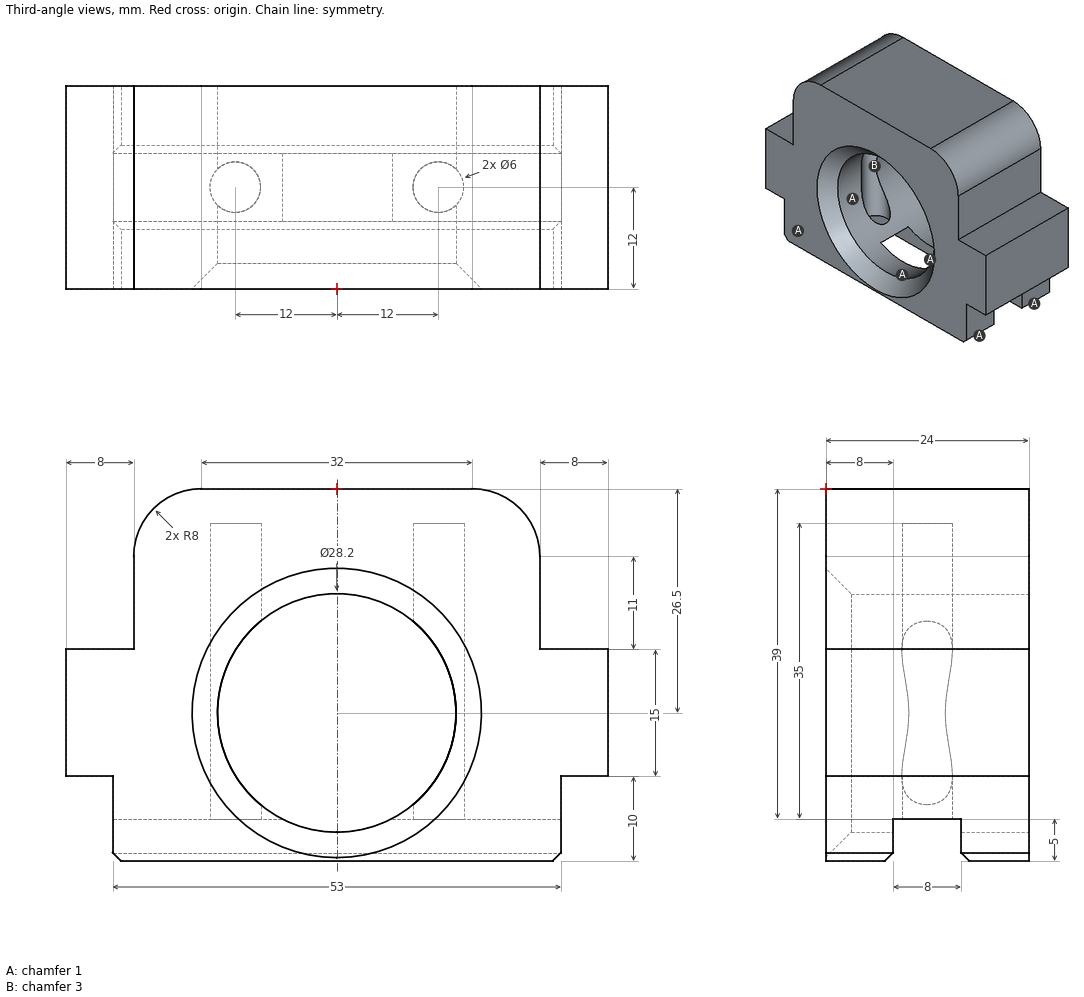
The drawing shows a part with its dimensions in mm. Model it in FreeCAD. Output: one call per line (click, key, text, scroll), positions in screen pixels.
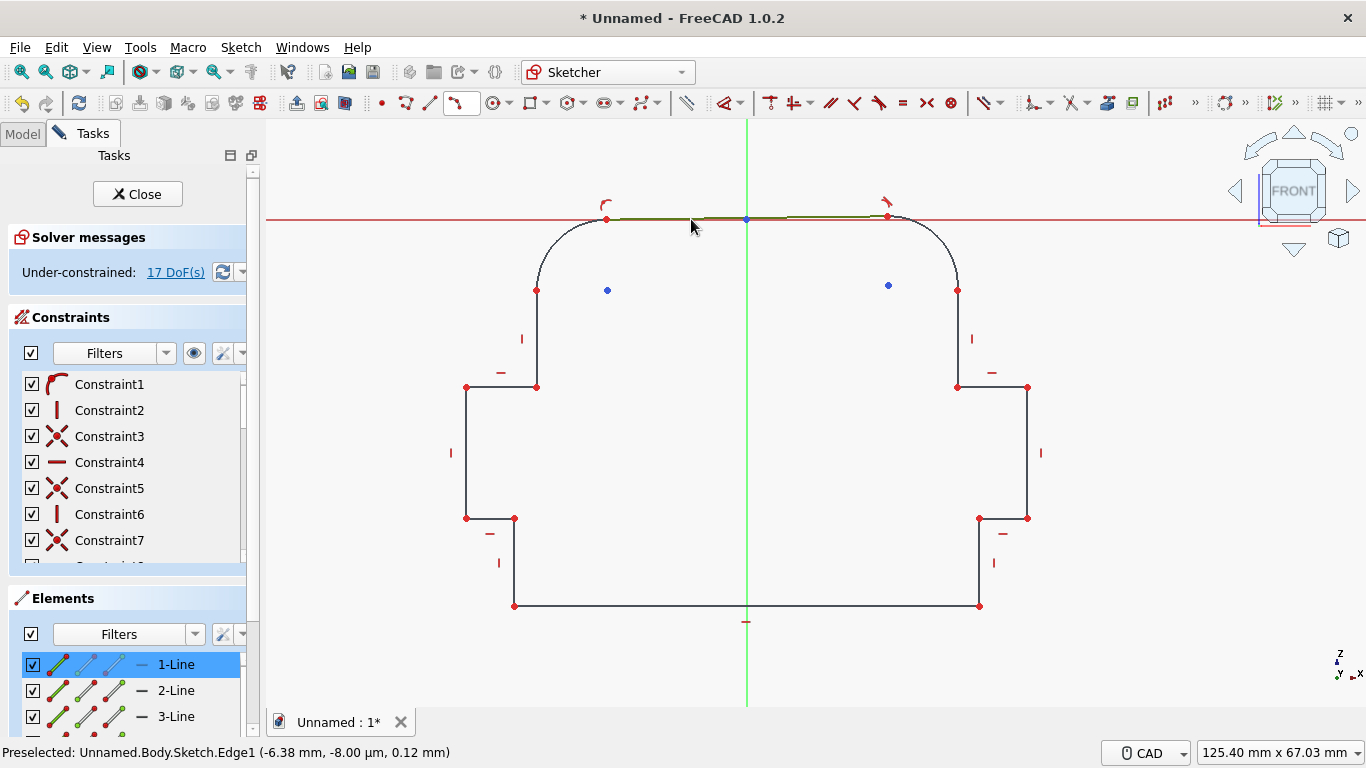
click(544, 259)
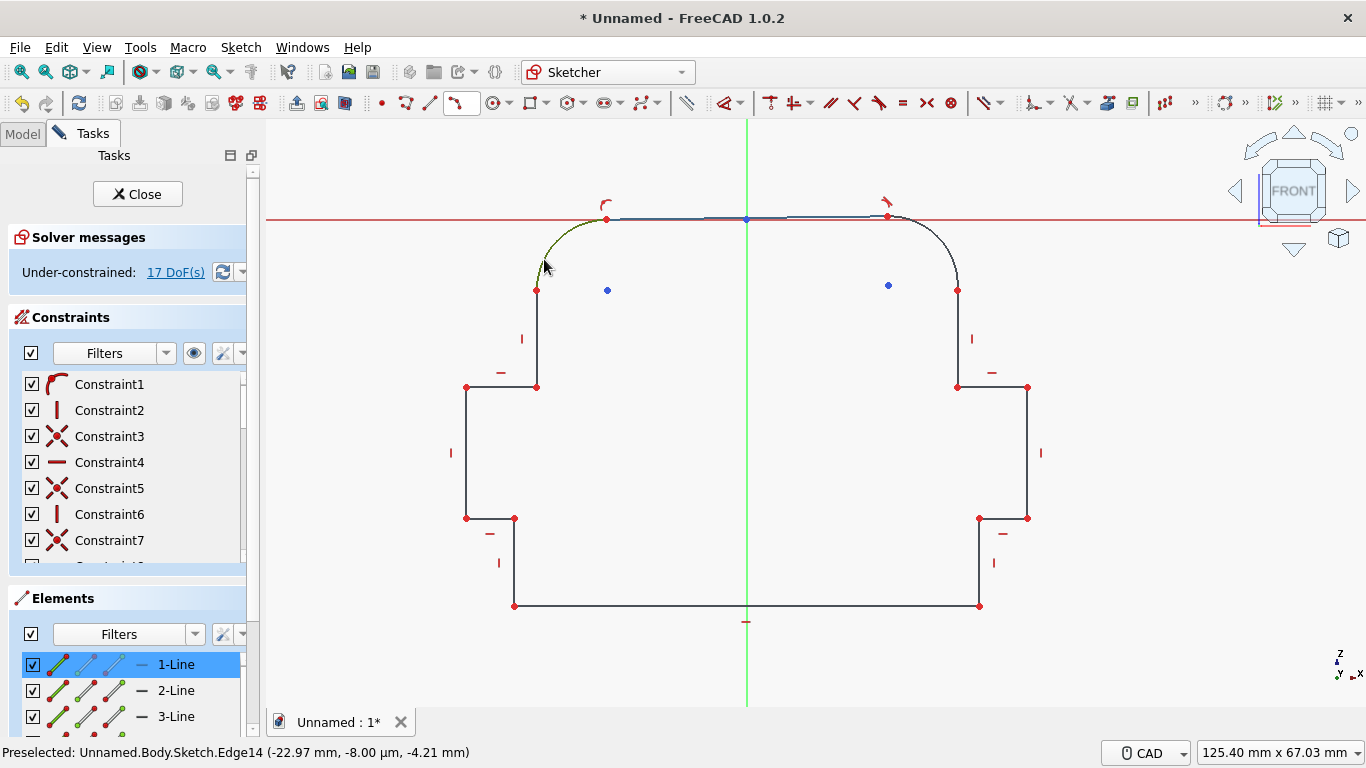
click(880, 104)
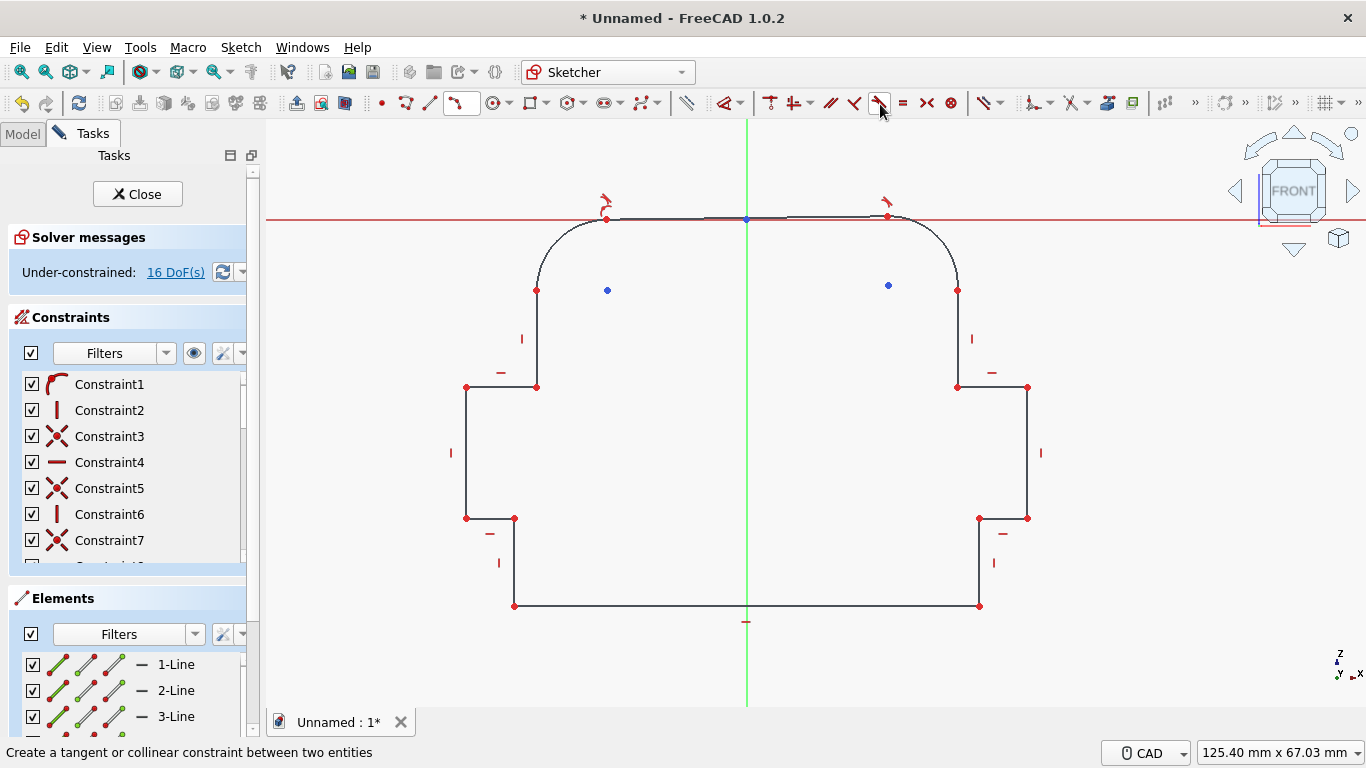
click(958, 319)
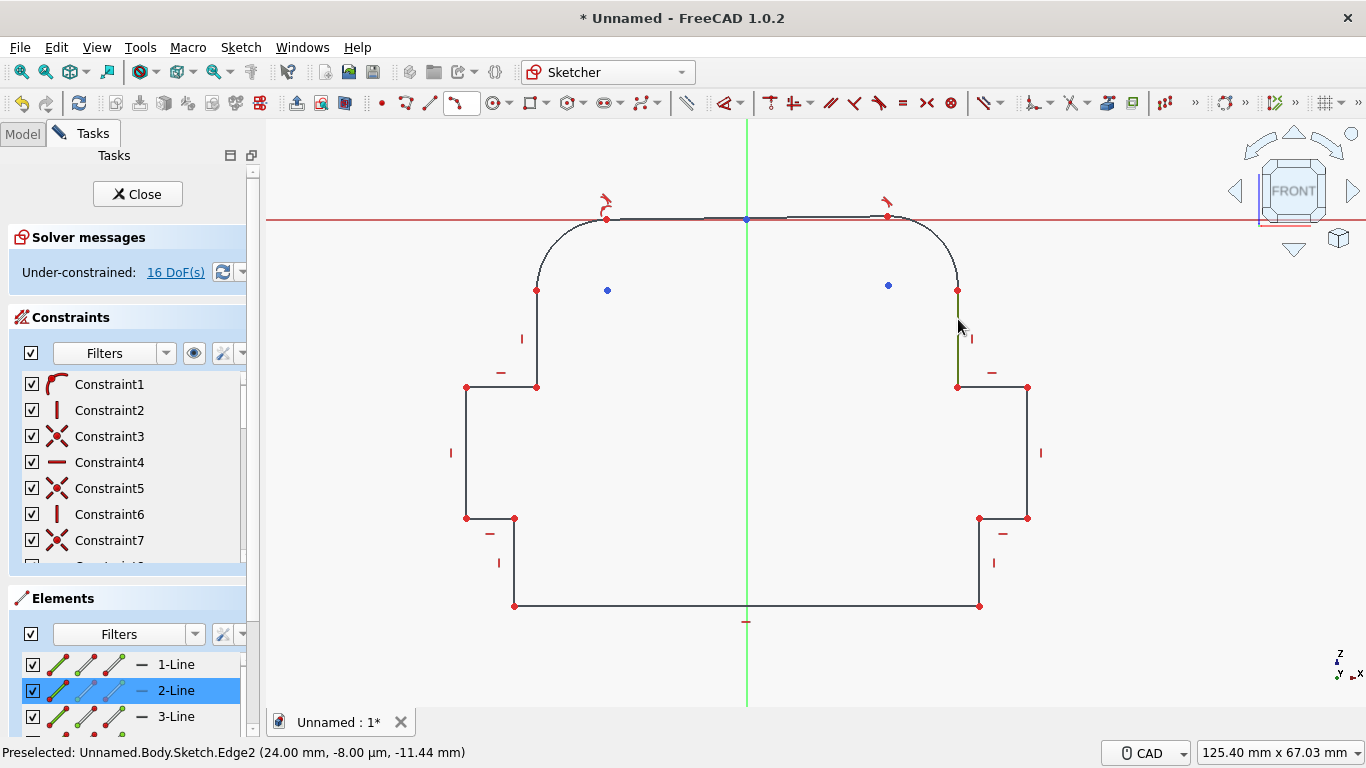
click(952, 257)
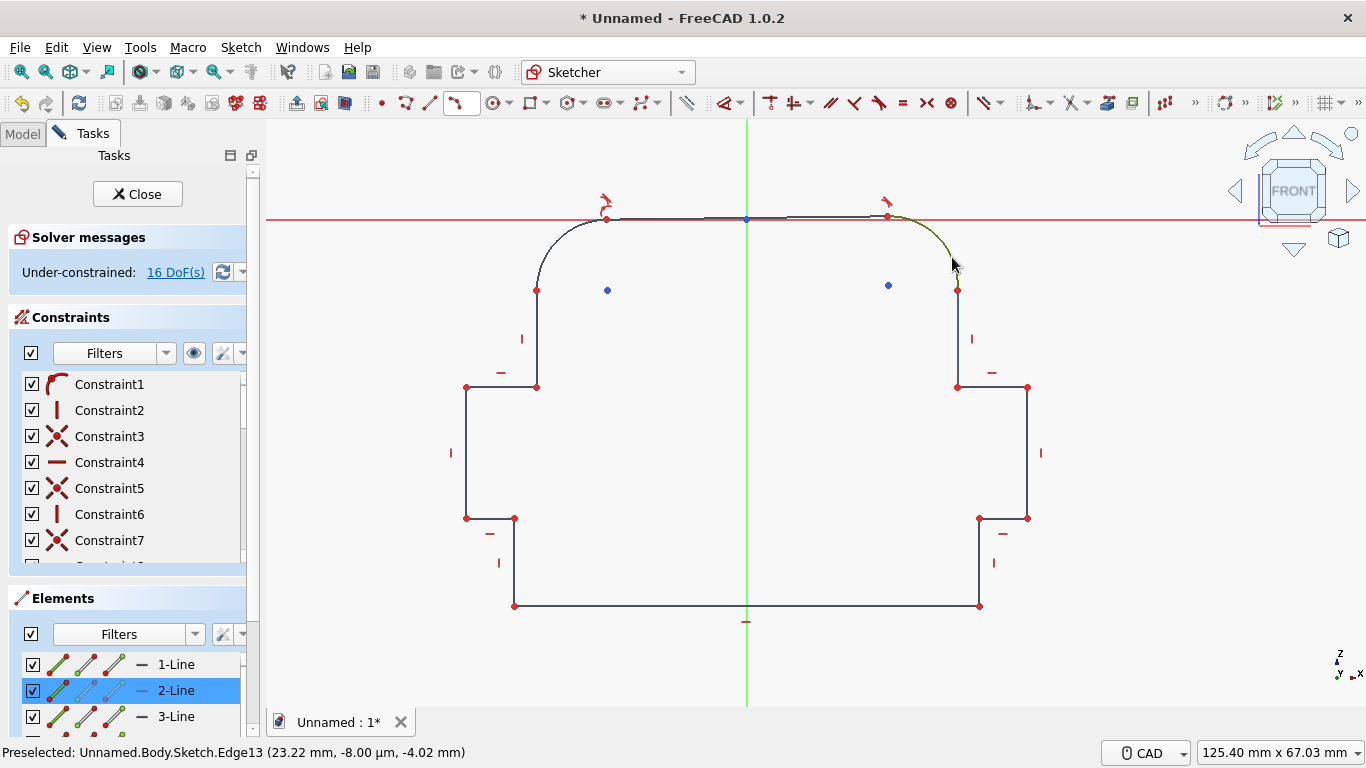
click(880, 104)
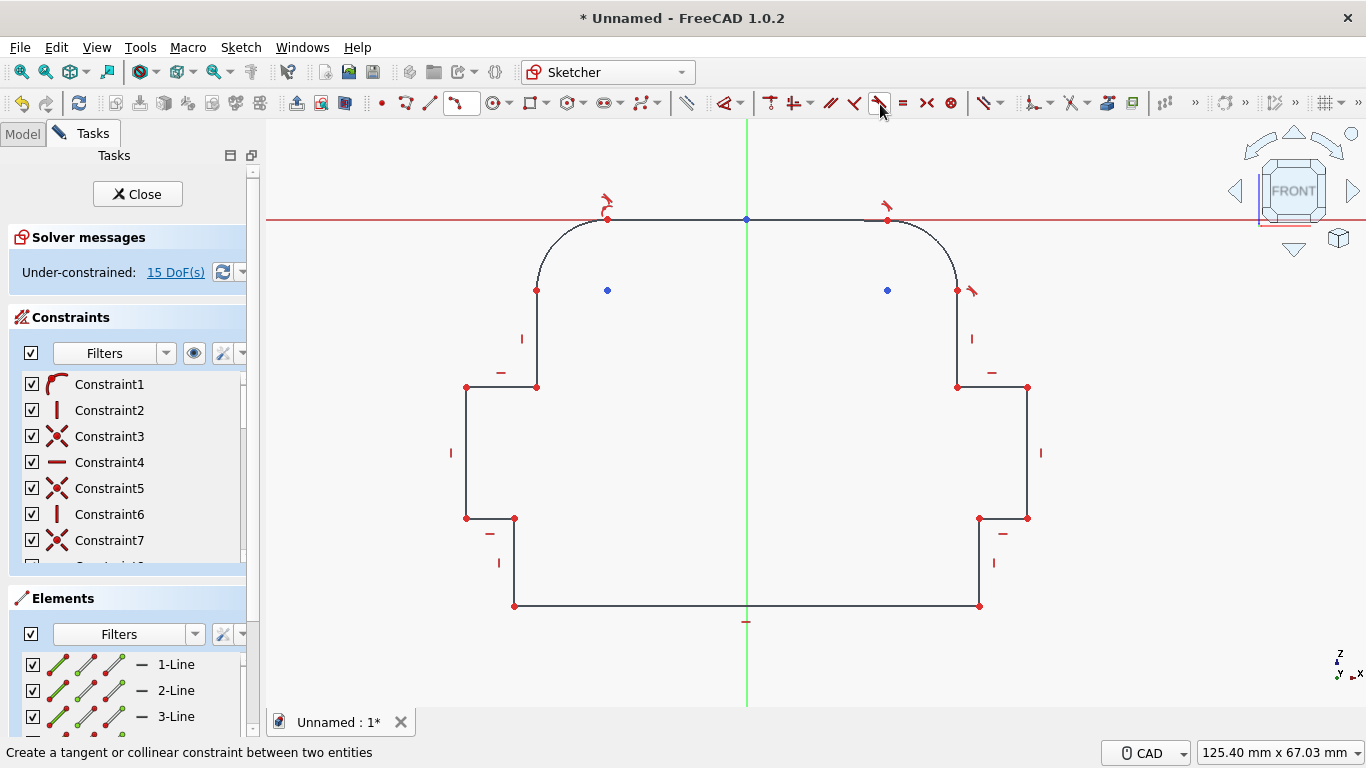
click(537, 358)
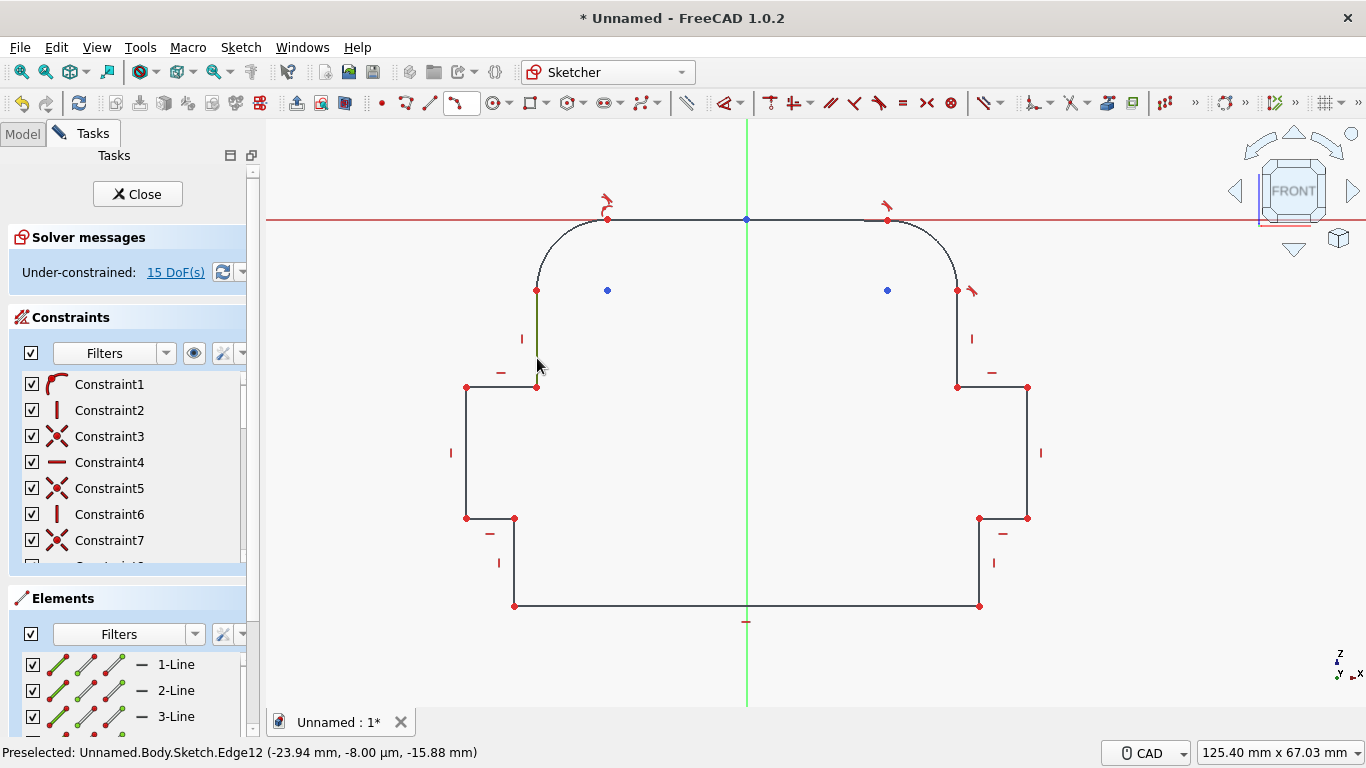
click(545, 258)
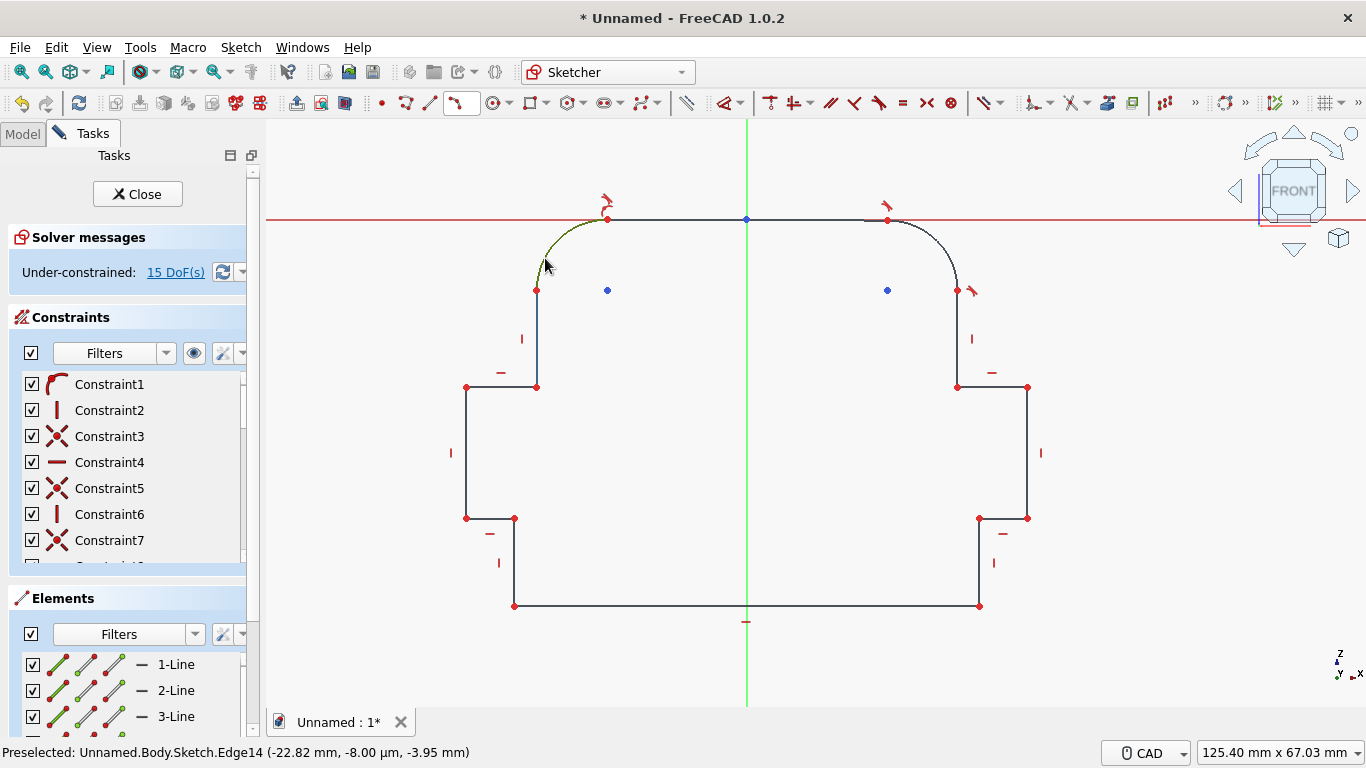
click(880, 104)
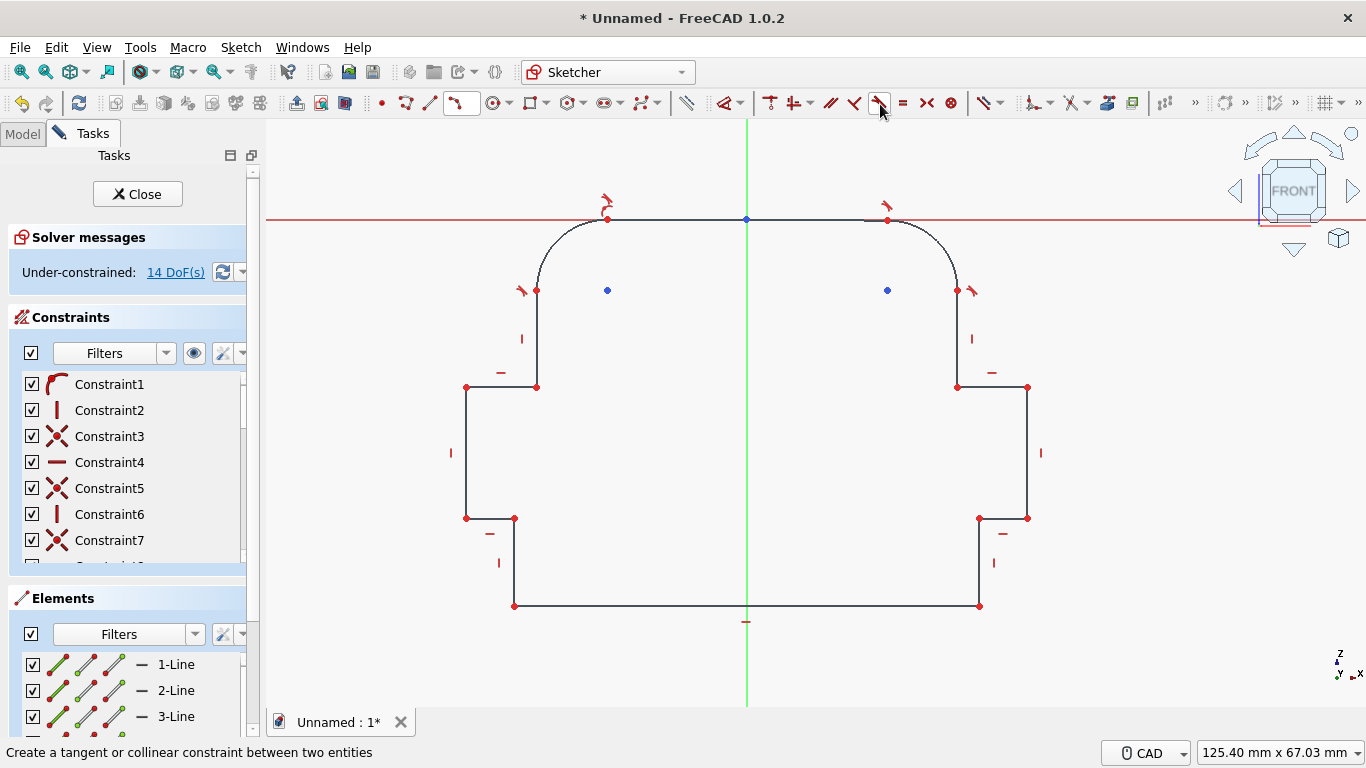
click(692, 220)